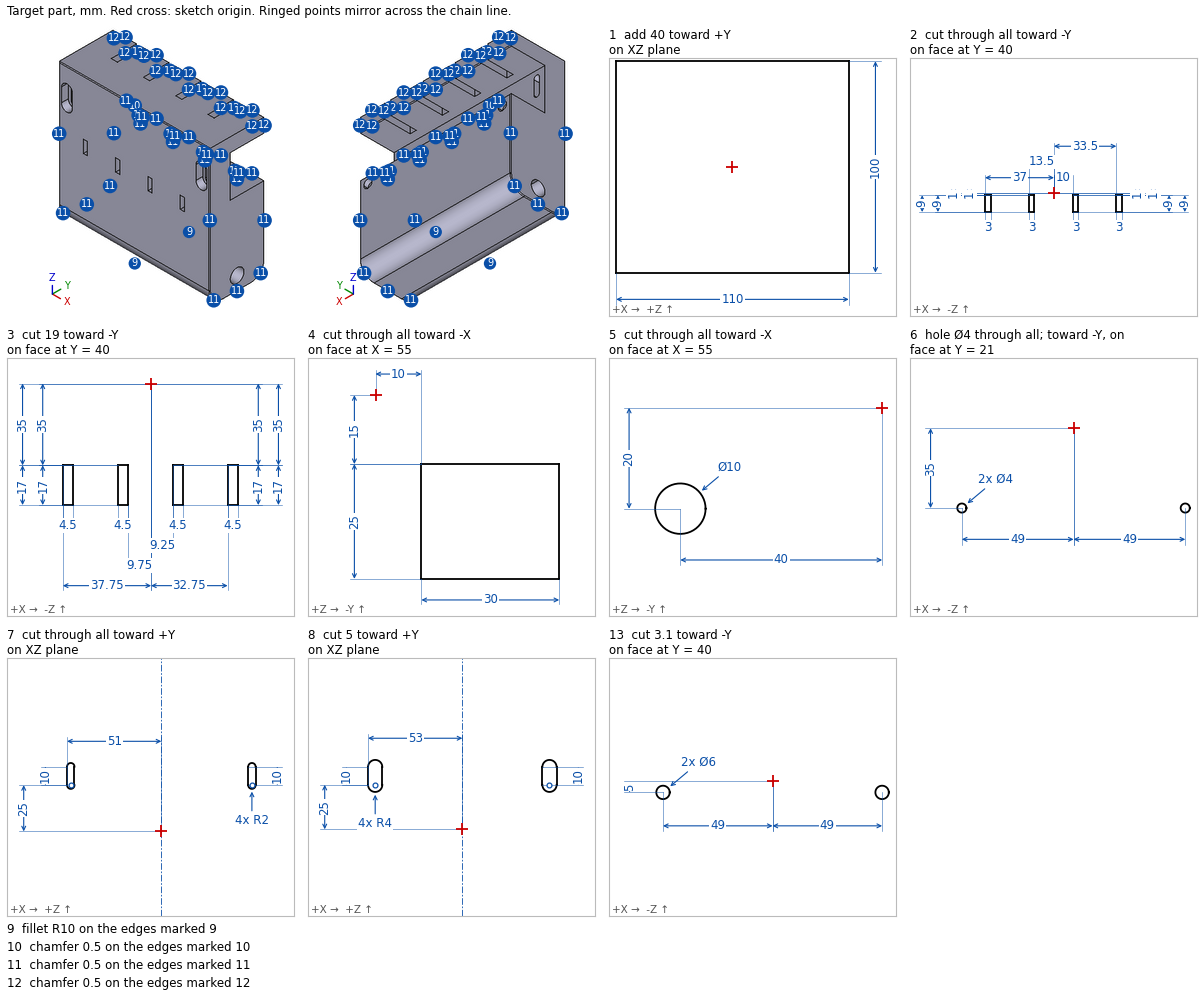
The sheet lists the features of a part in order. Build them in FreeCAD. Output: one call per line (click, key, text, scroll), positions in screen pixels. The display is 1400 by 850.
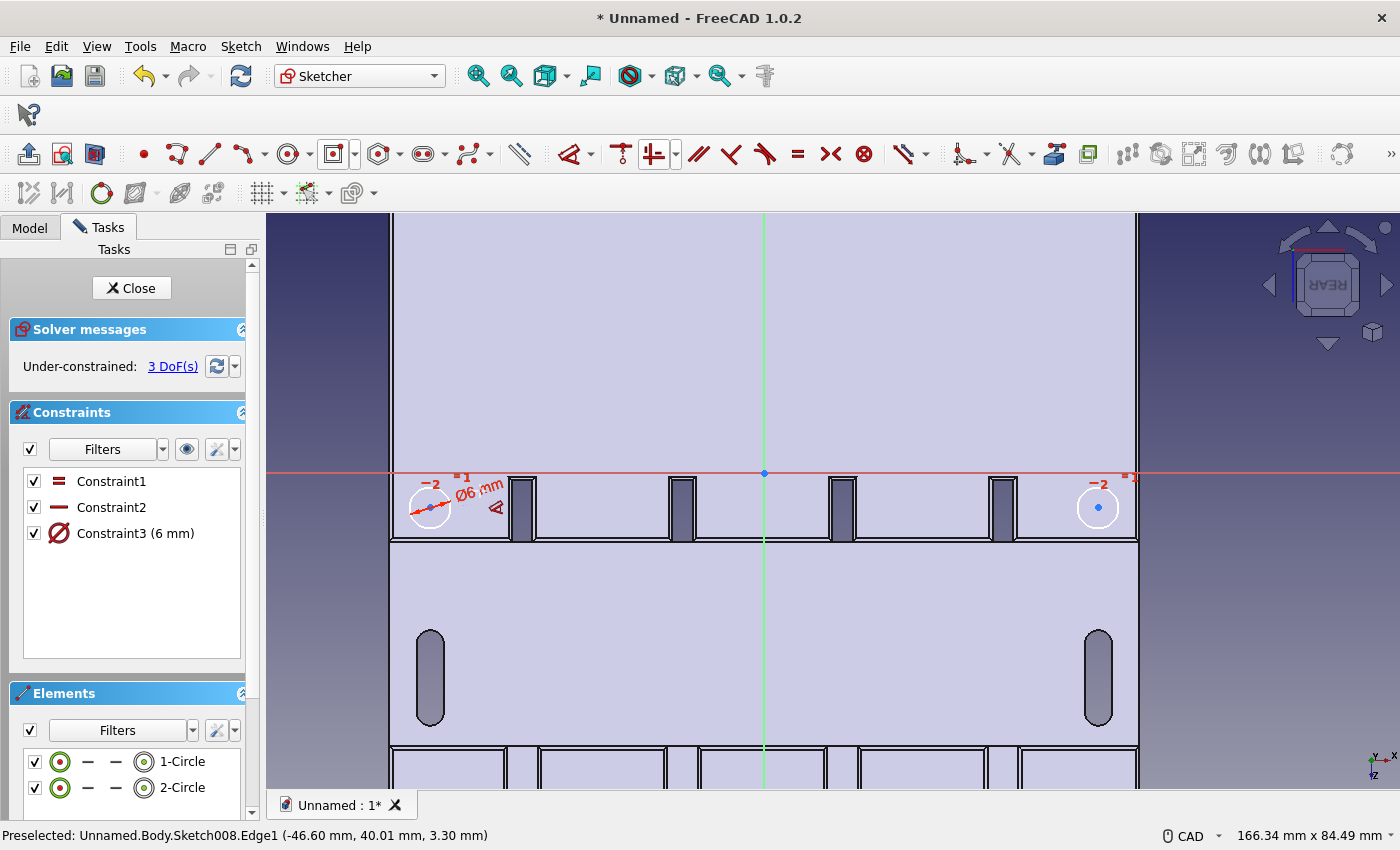
click(430, 508)
click(396, 491)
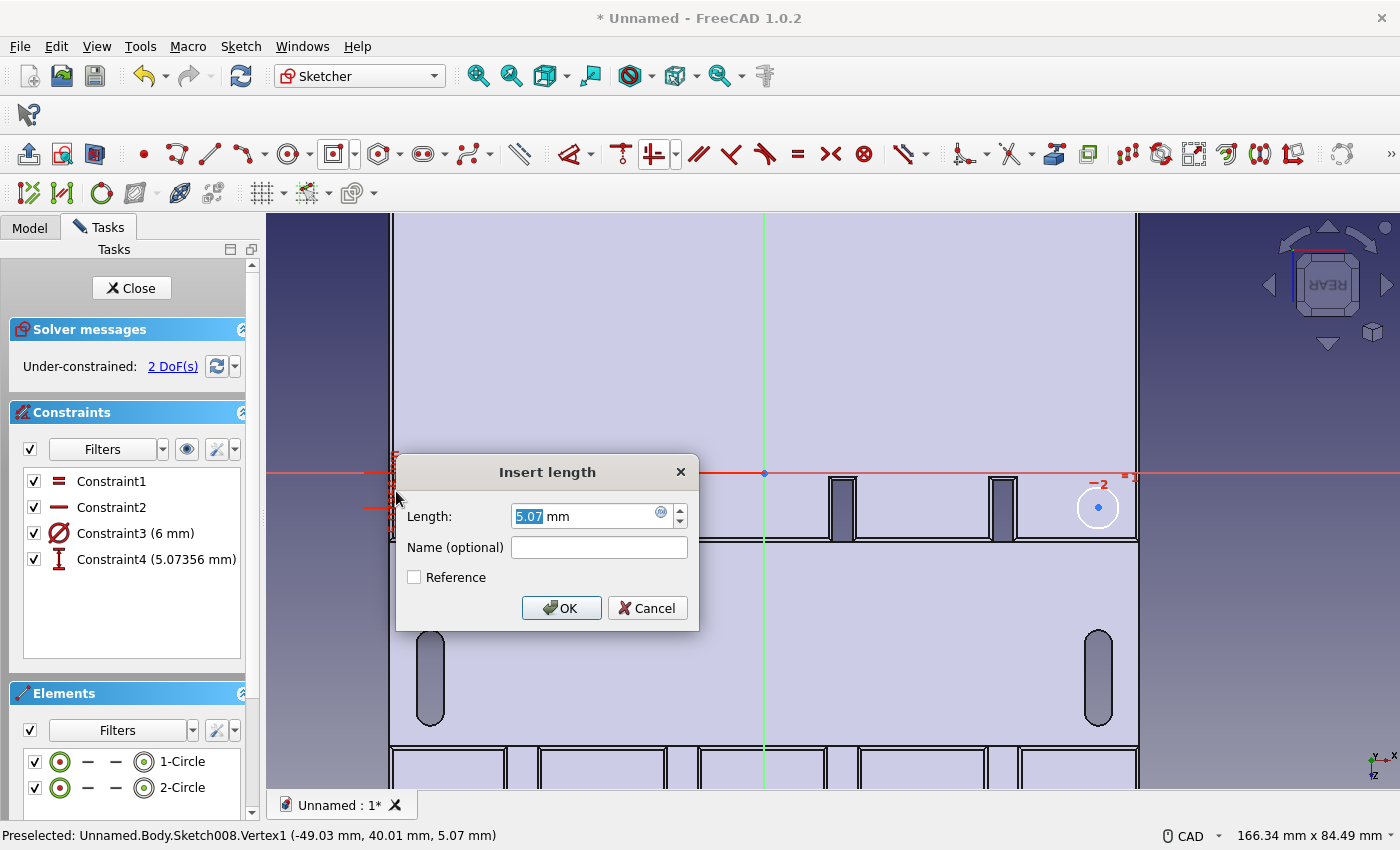
text(5)
key(Return)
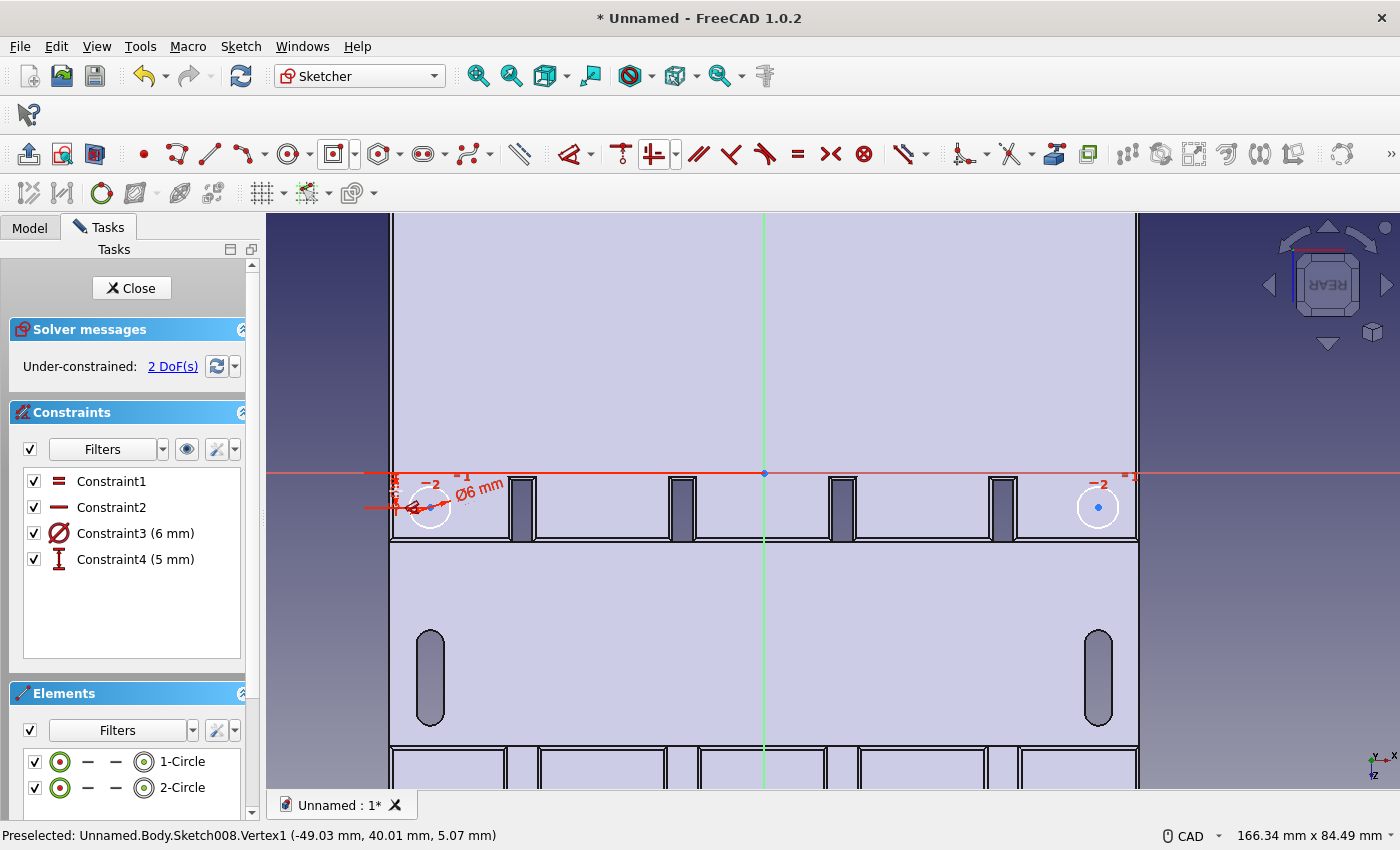
click(430, 507)
click(597, 439)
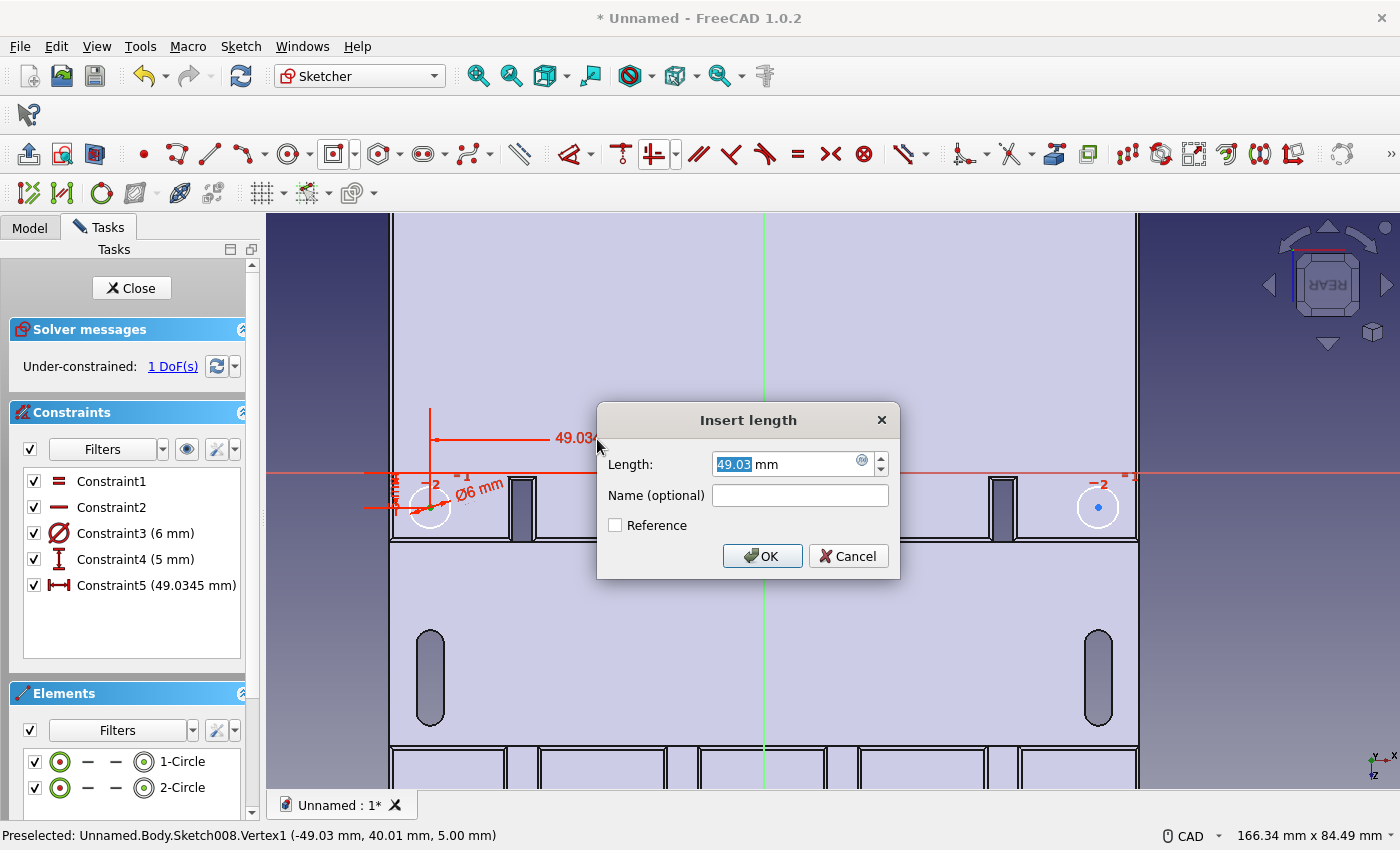
text(49)
key(Return)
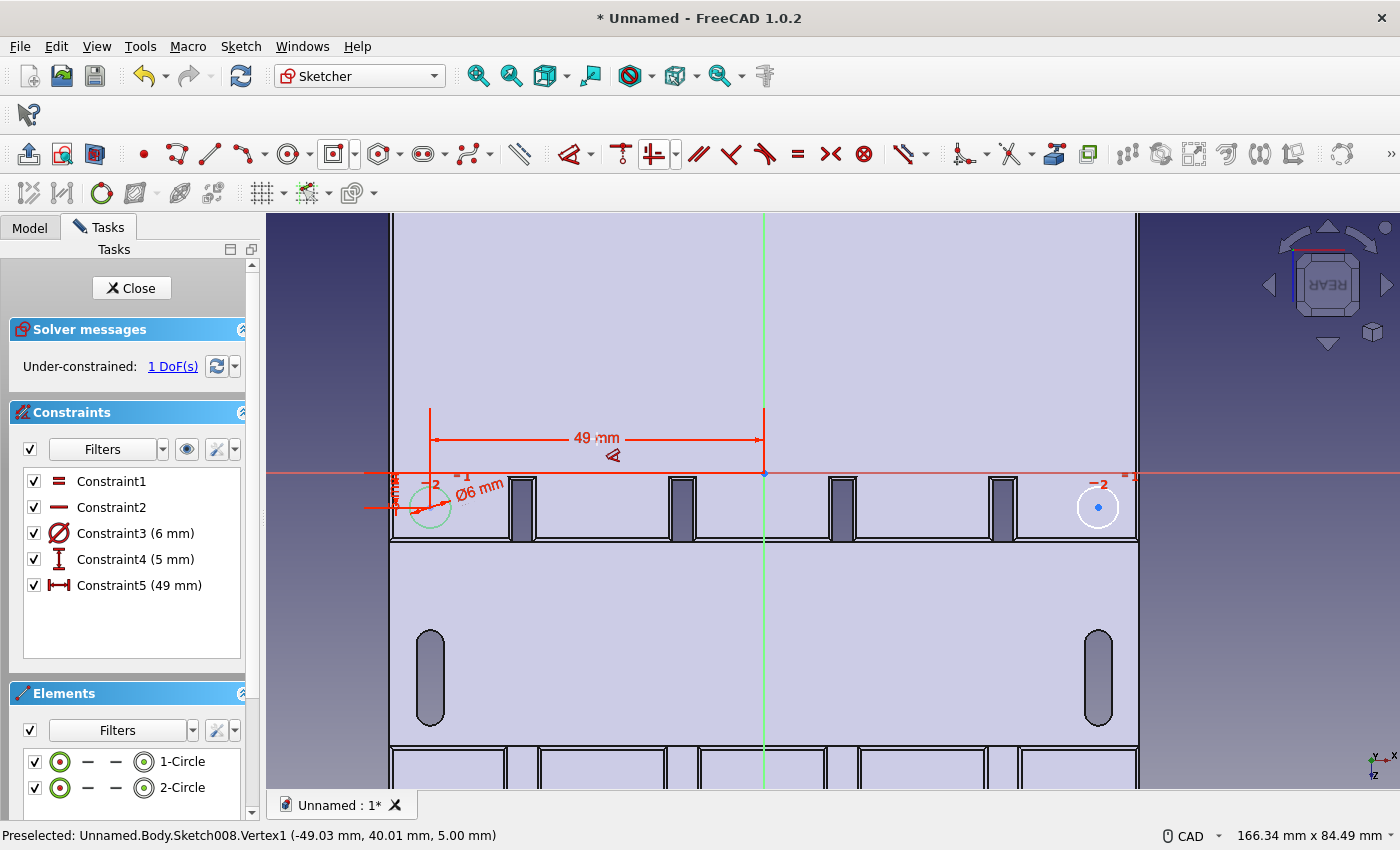
click(1098, 507)
click(931, 439)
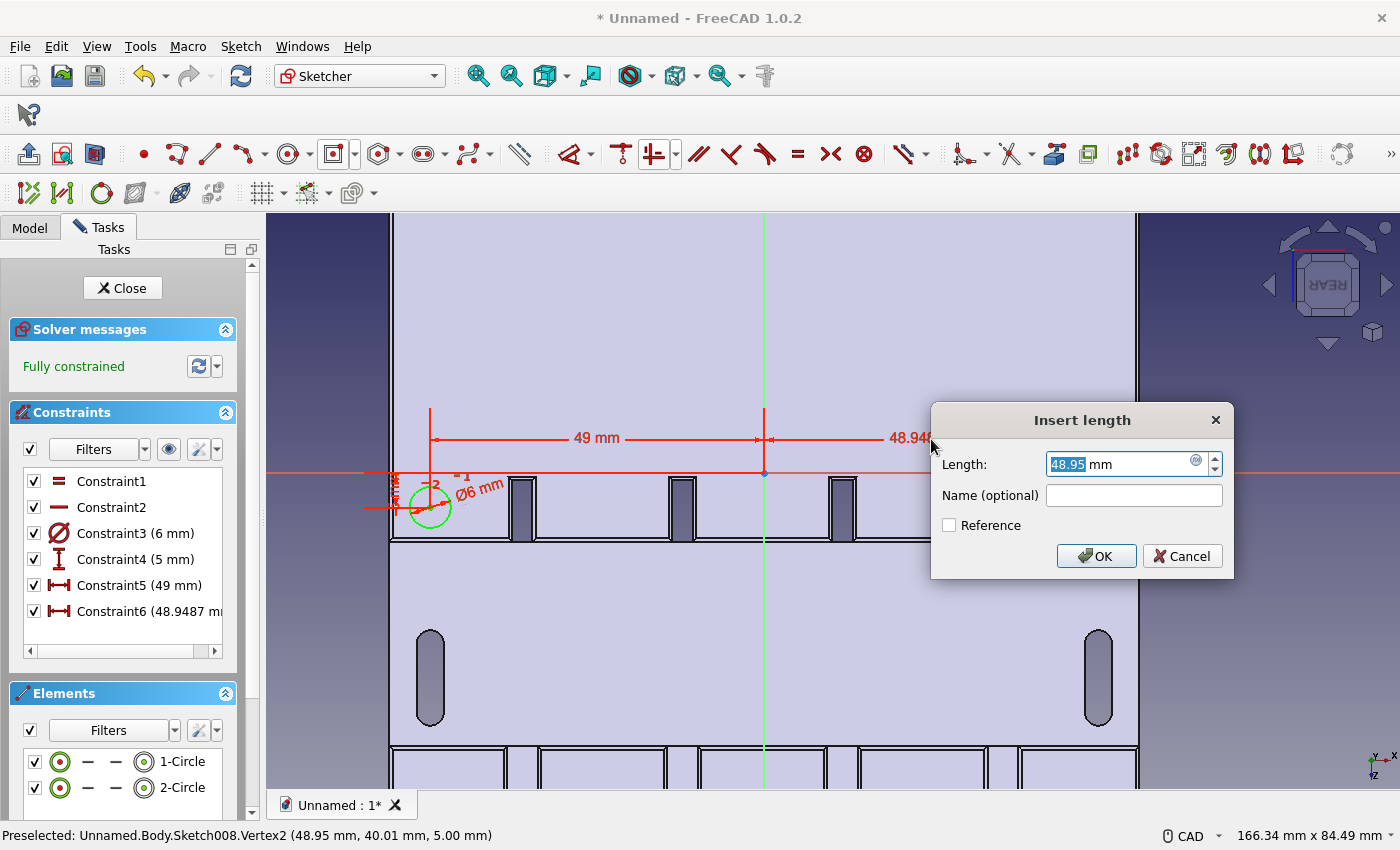
text(49)
key(Return)
key(Escape)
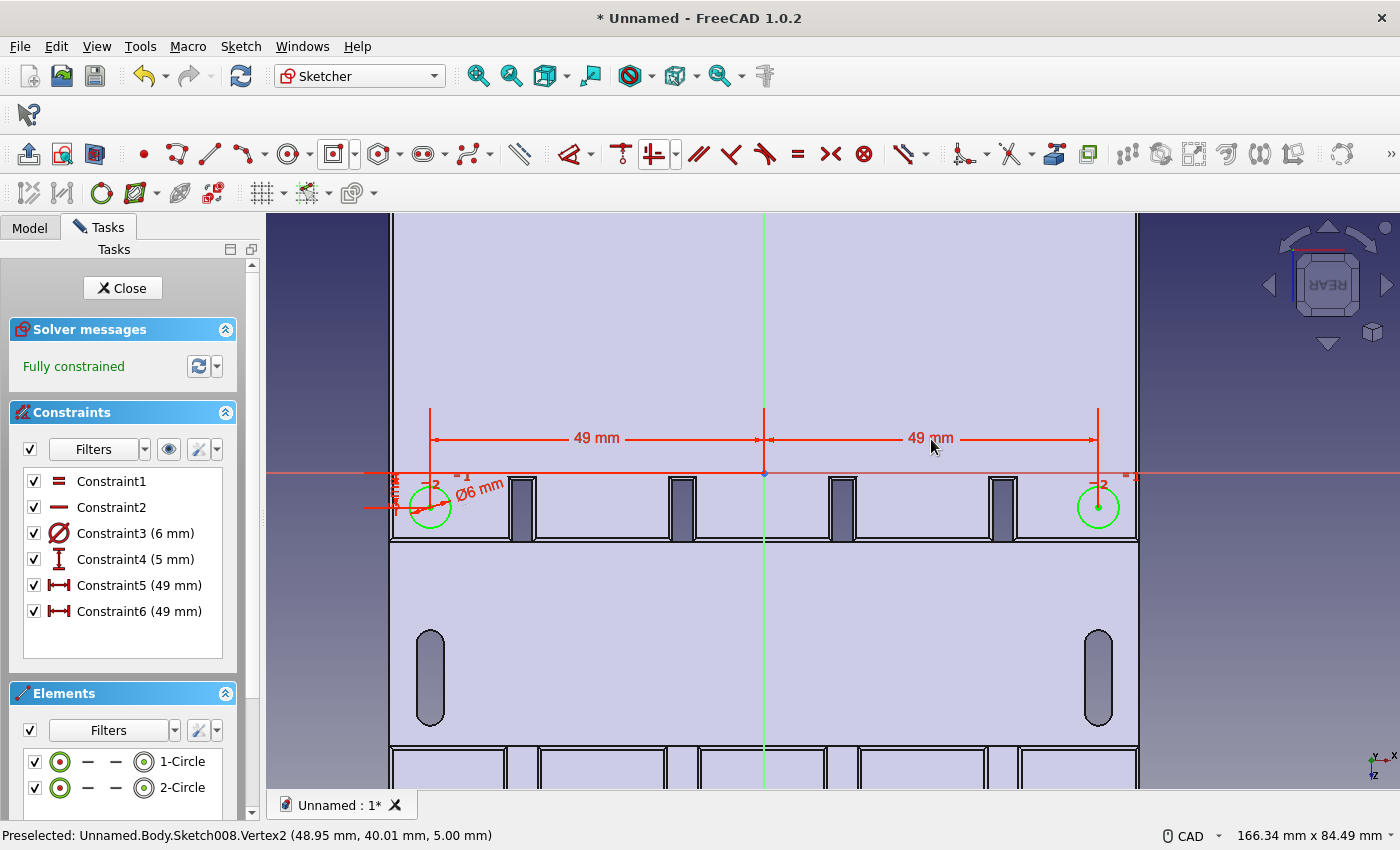
click(123, 288)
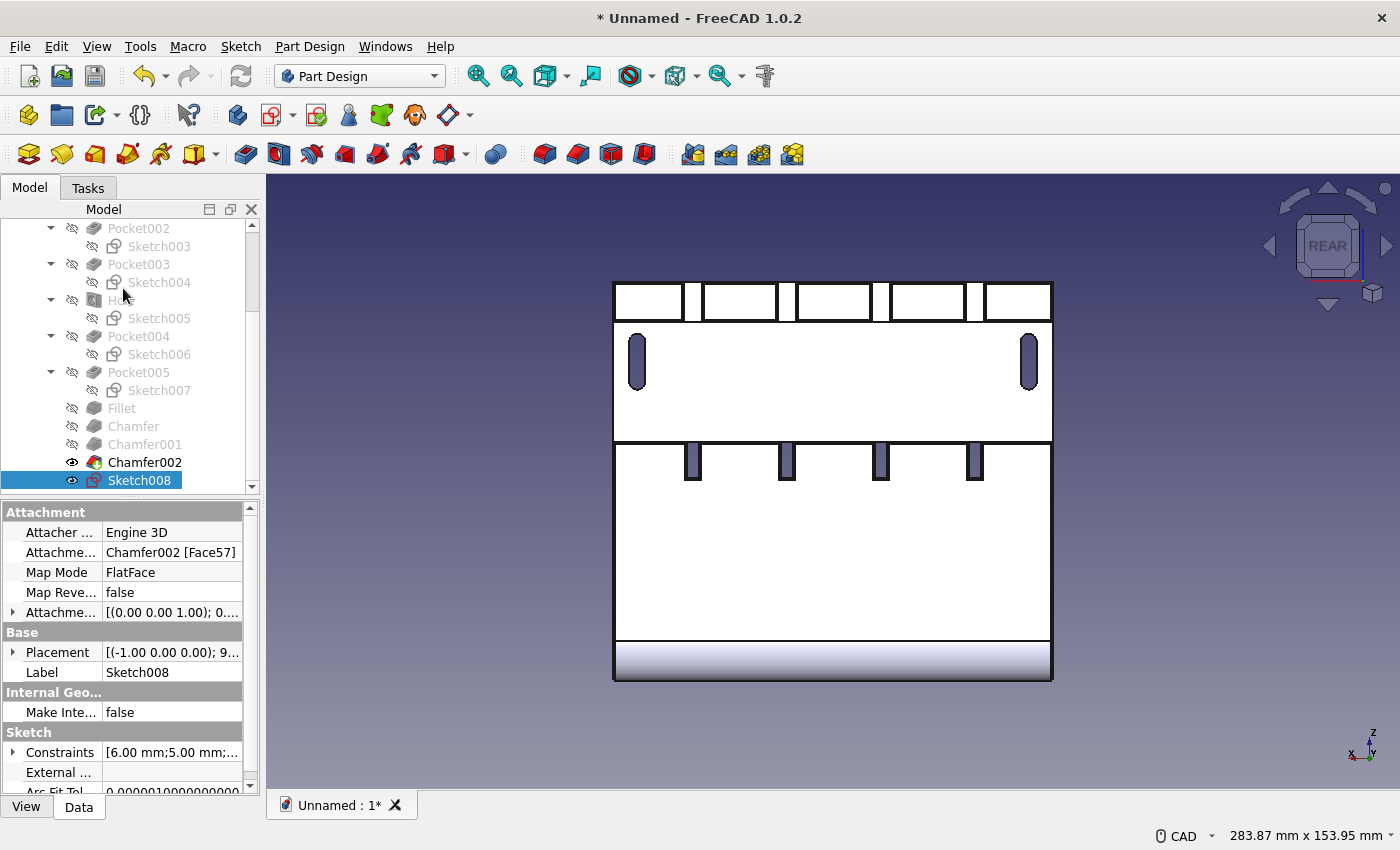
click(246, 154)